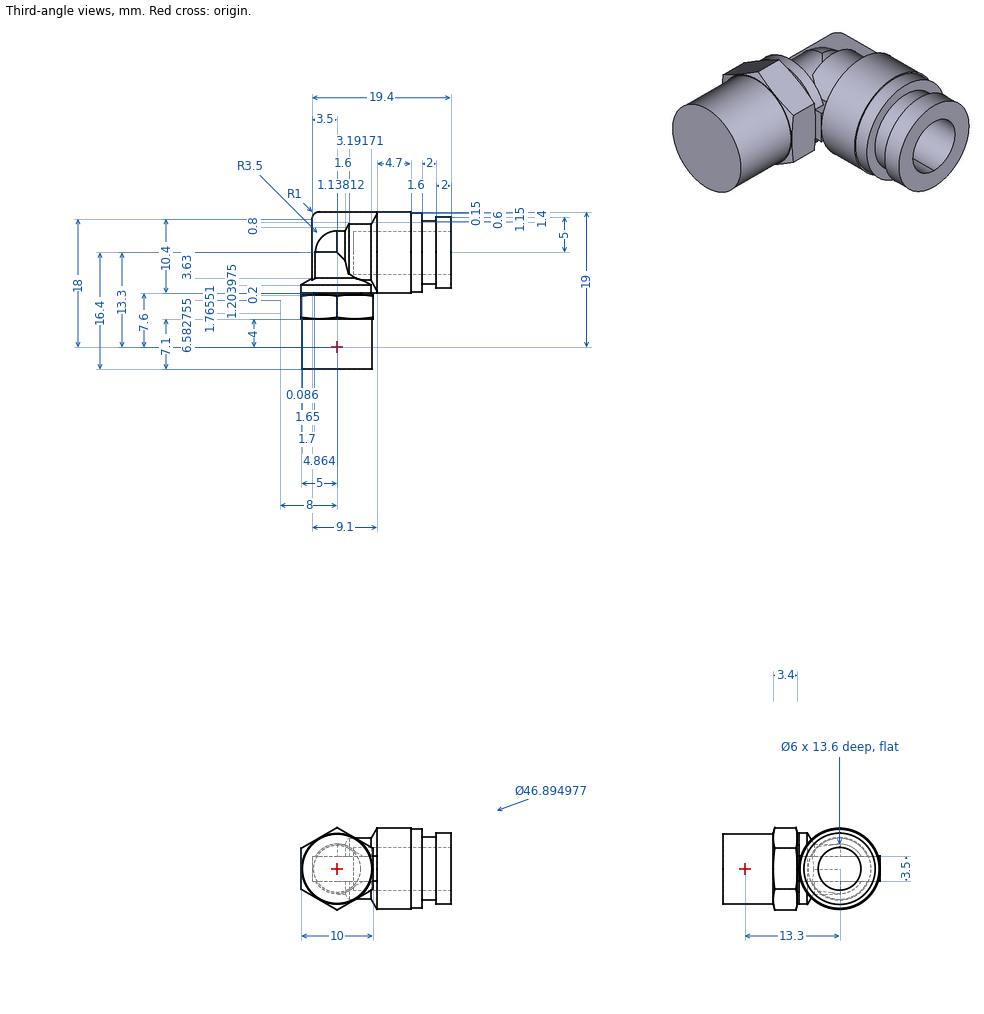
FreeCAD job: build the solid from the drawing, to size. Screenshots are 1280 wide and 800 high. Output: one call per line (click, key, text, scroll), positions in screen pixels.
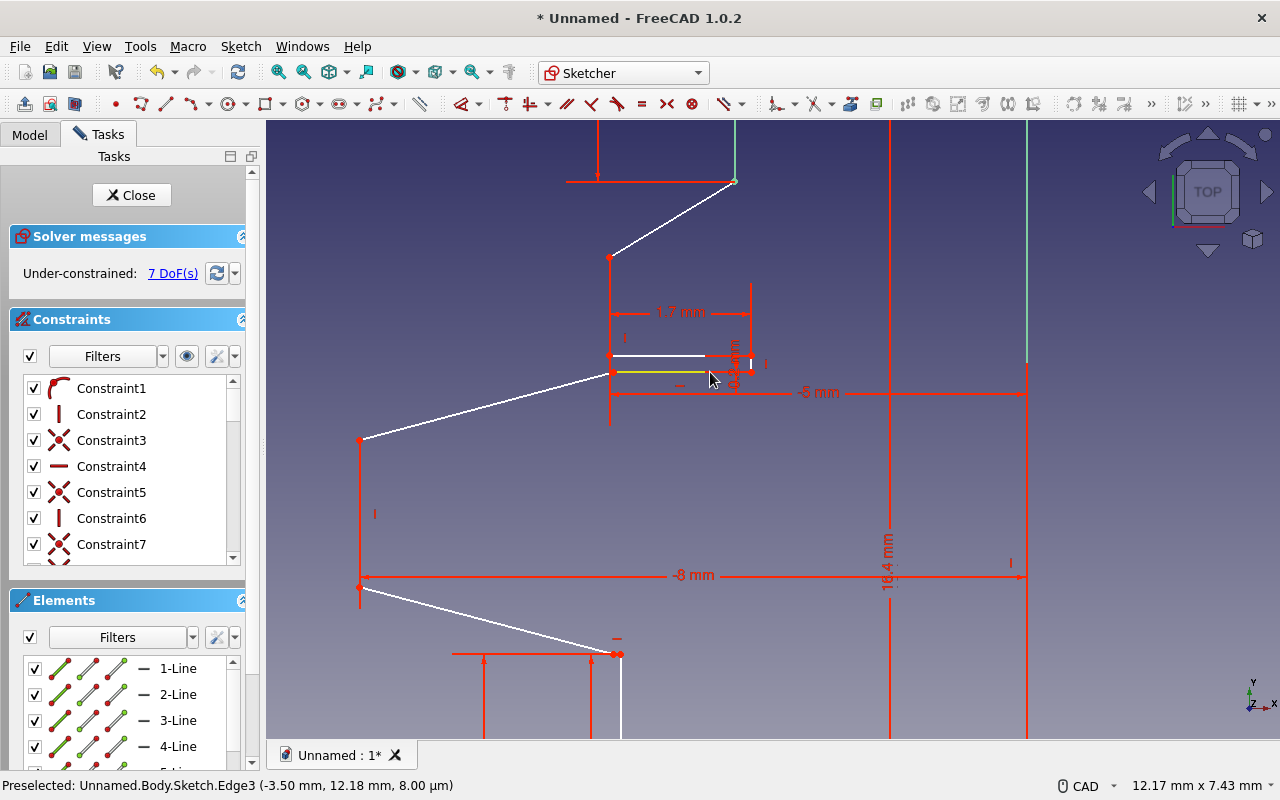
click(710, 372)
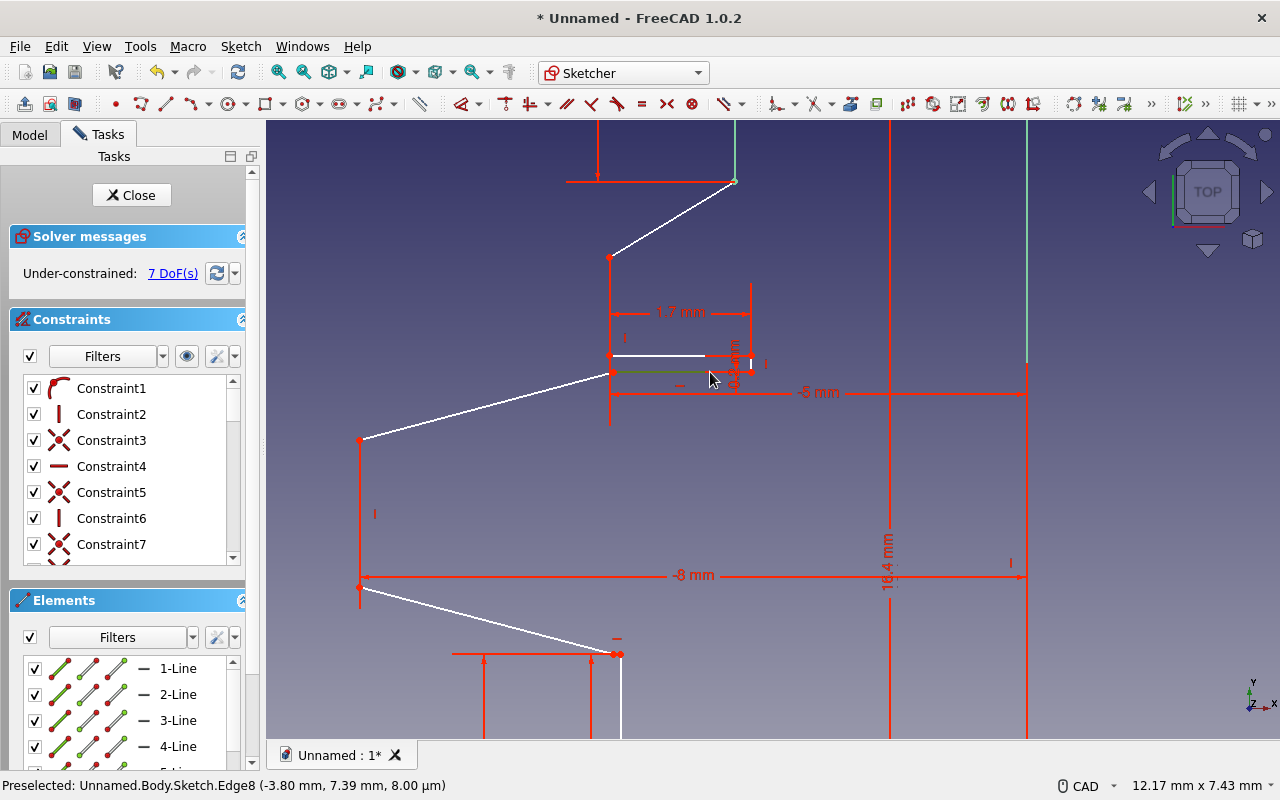
key(l)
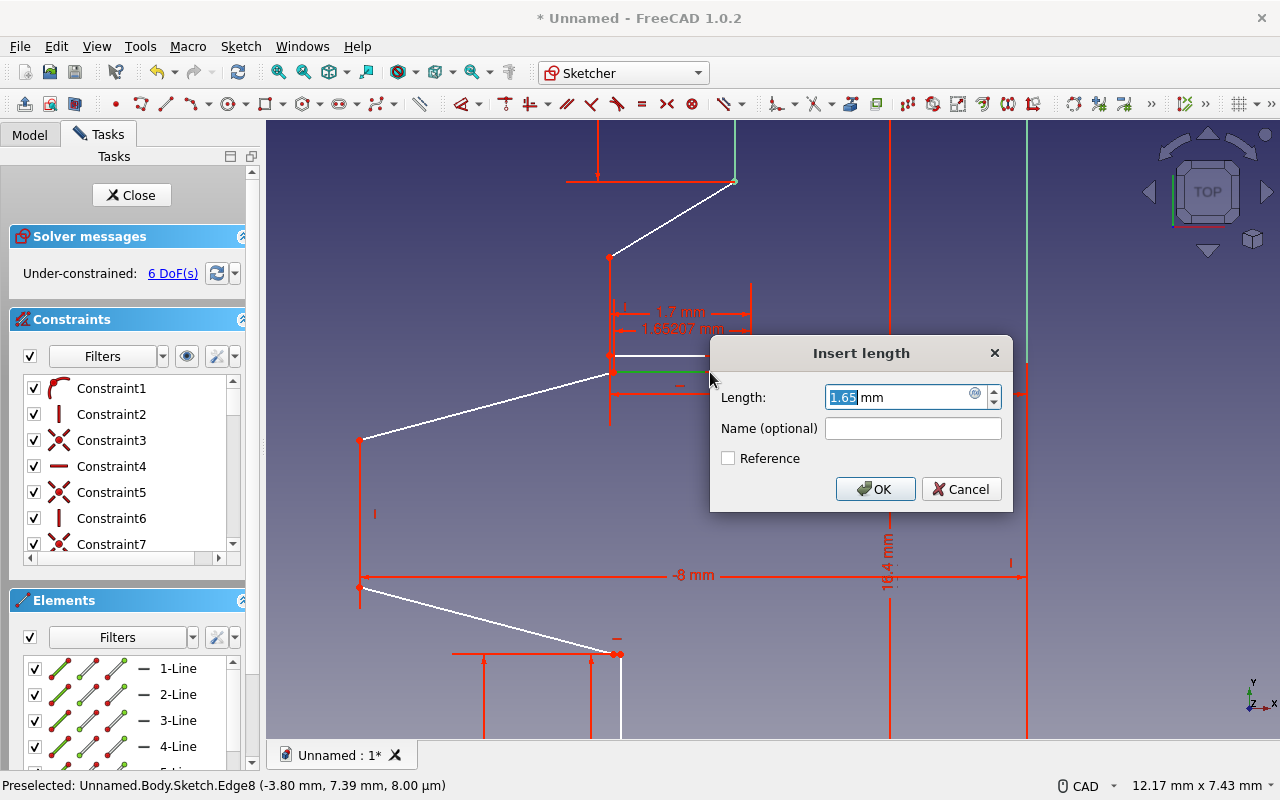
text(1.65)
key(Return)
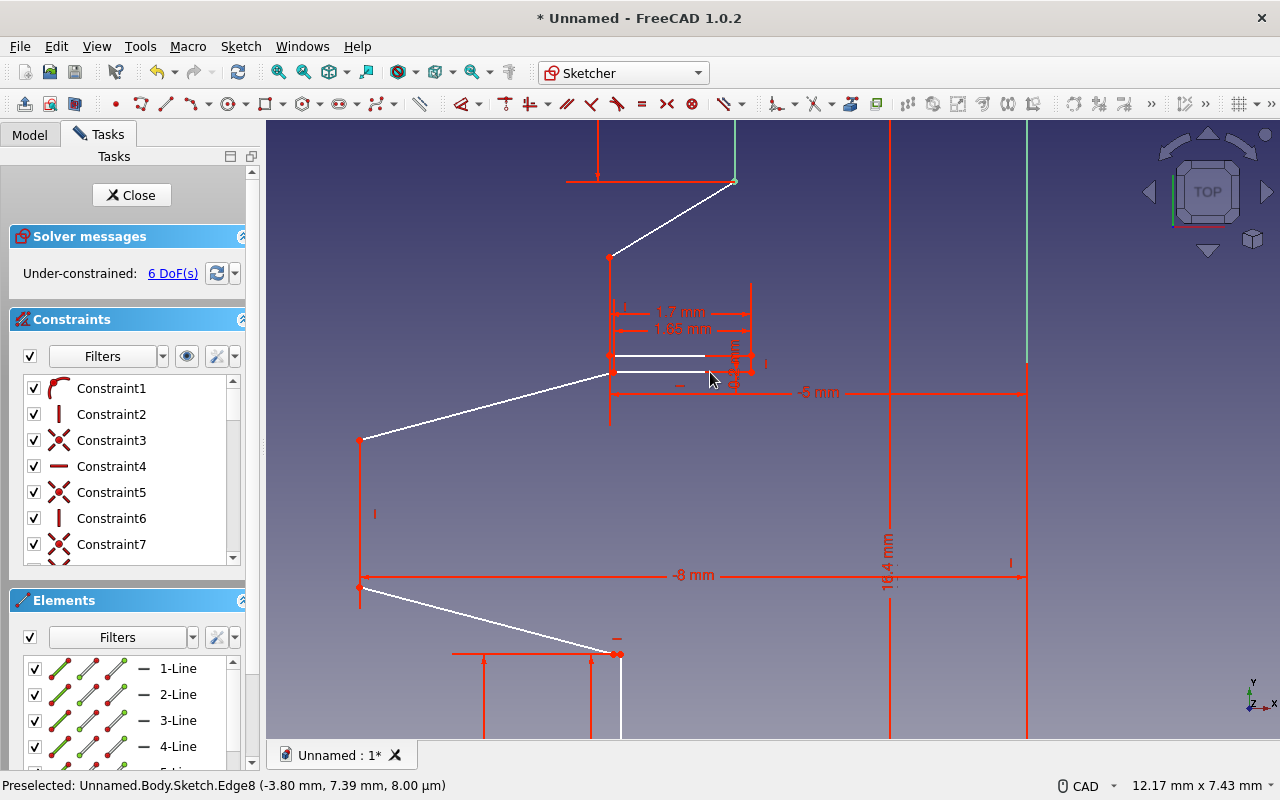
click(610, 356)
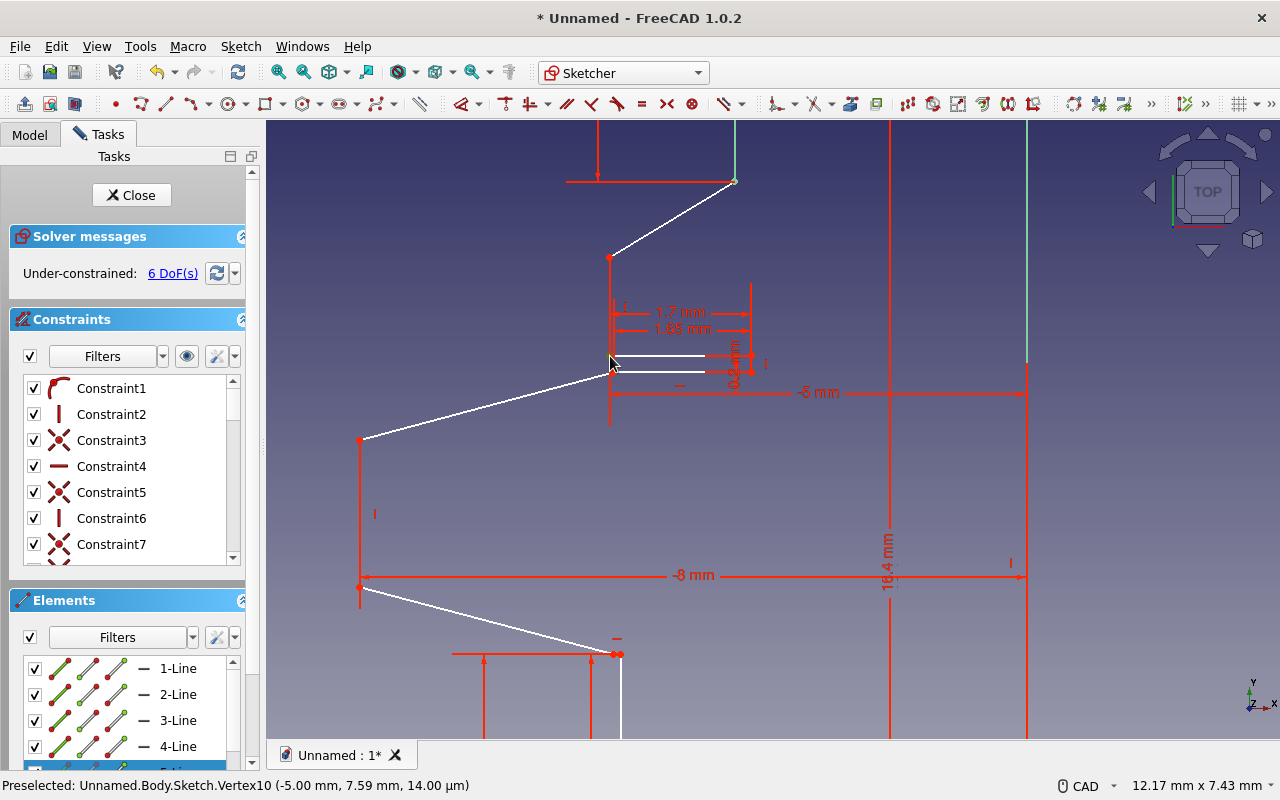
key(i)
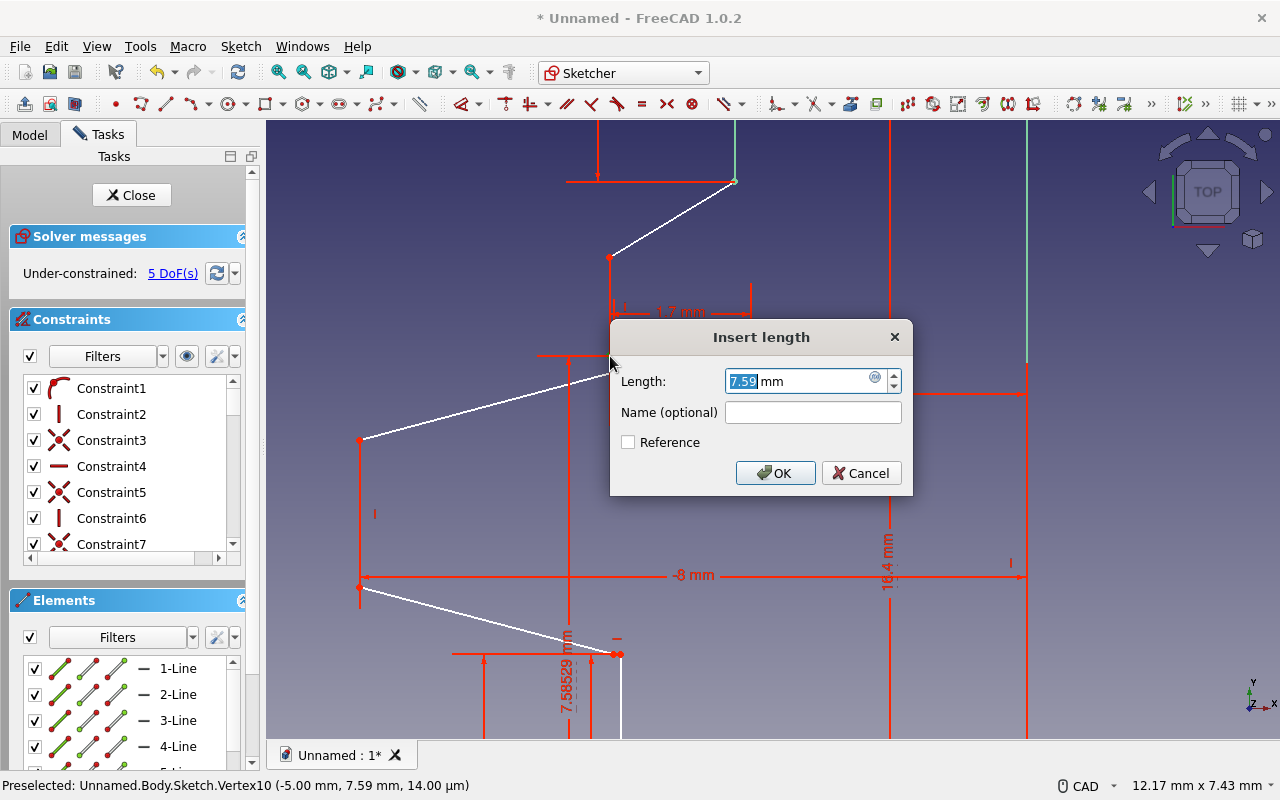
text(7.6)
key(Return)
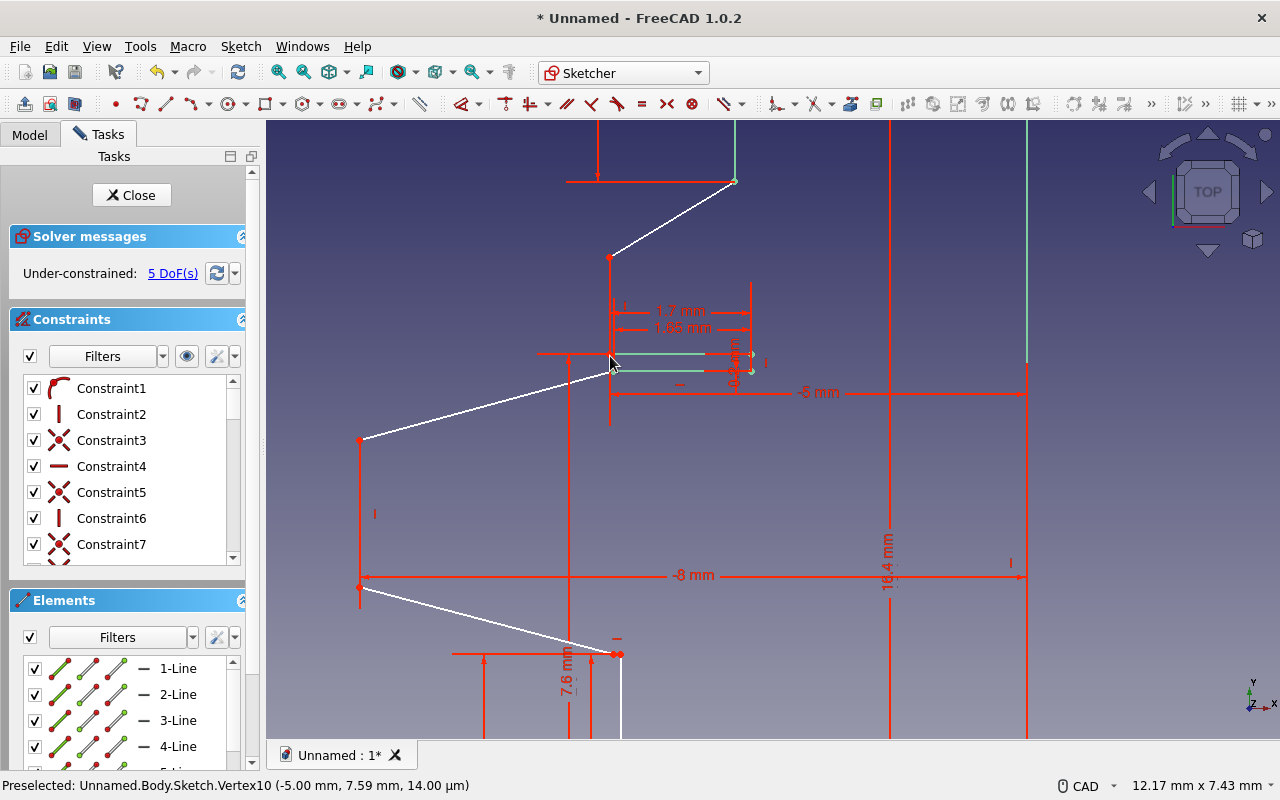
scroll(617, 654, up, 9)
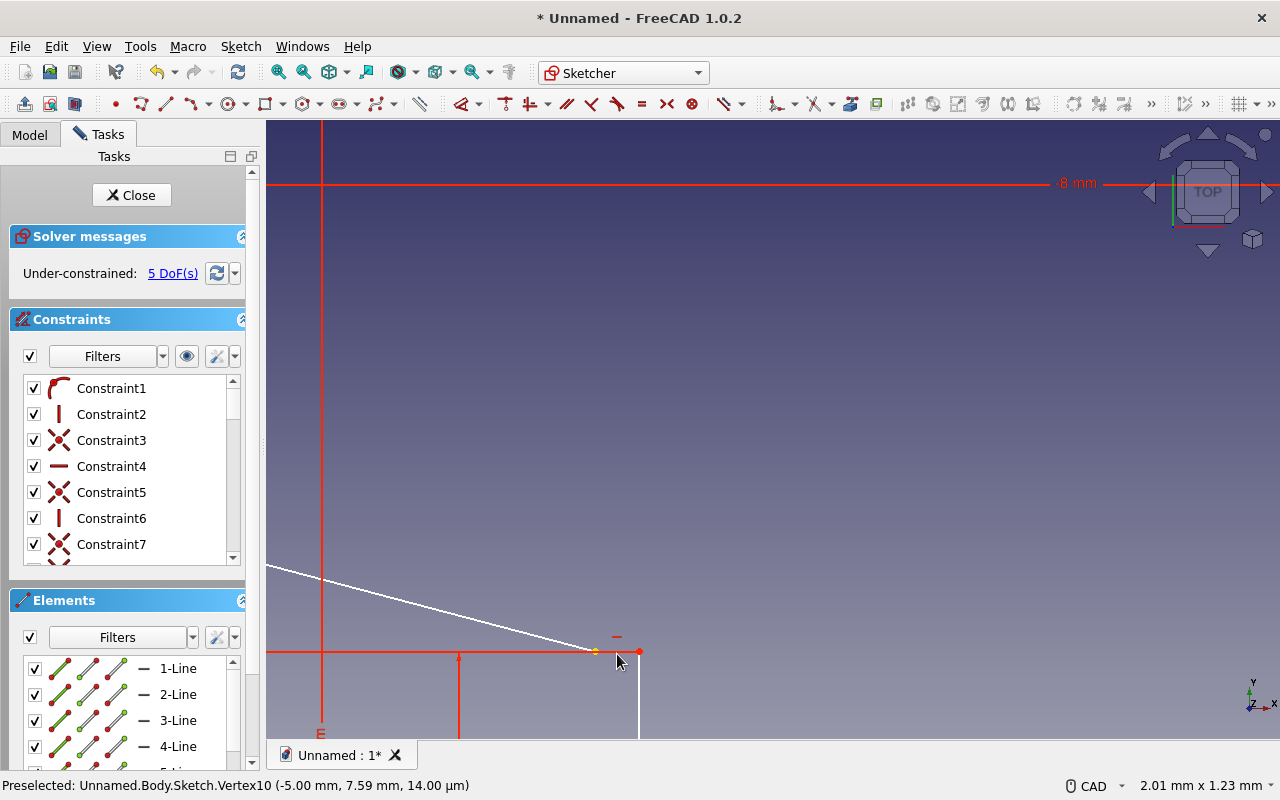
click(618, 652)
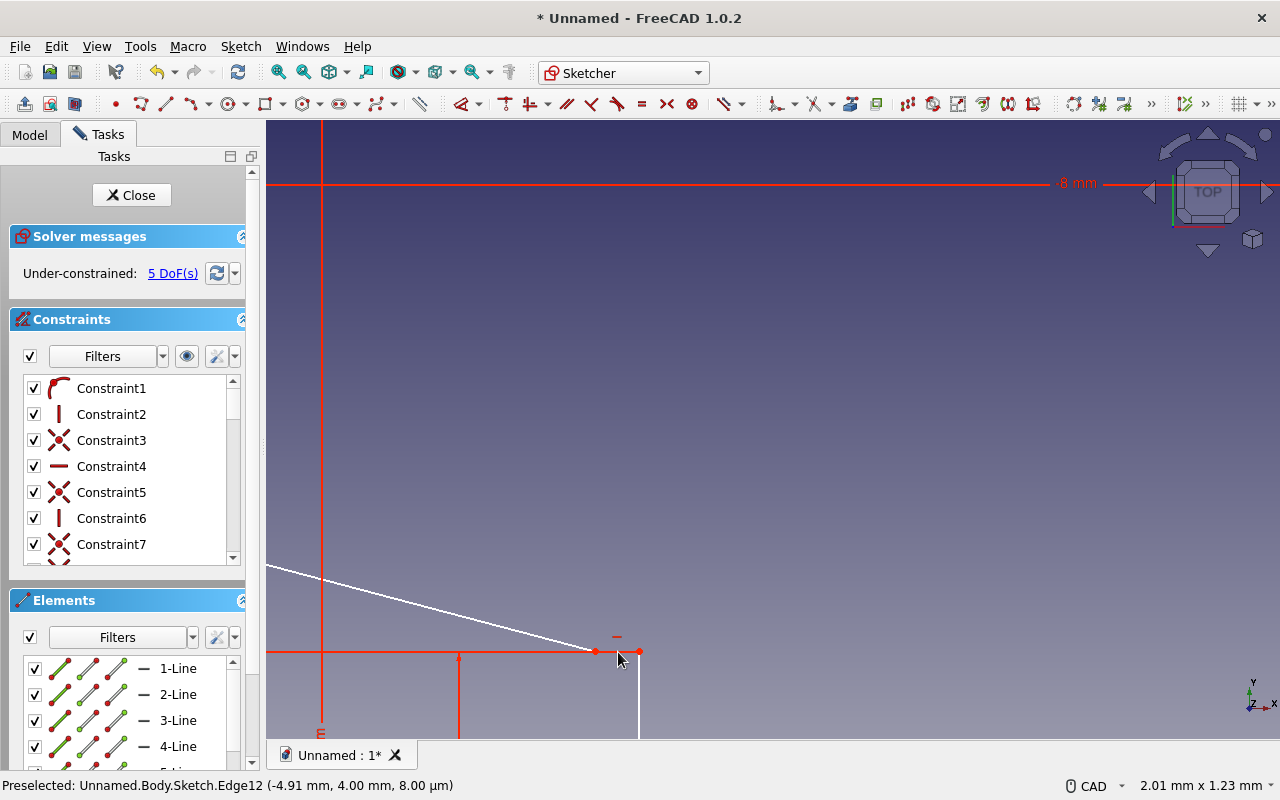
key(l)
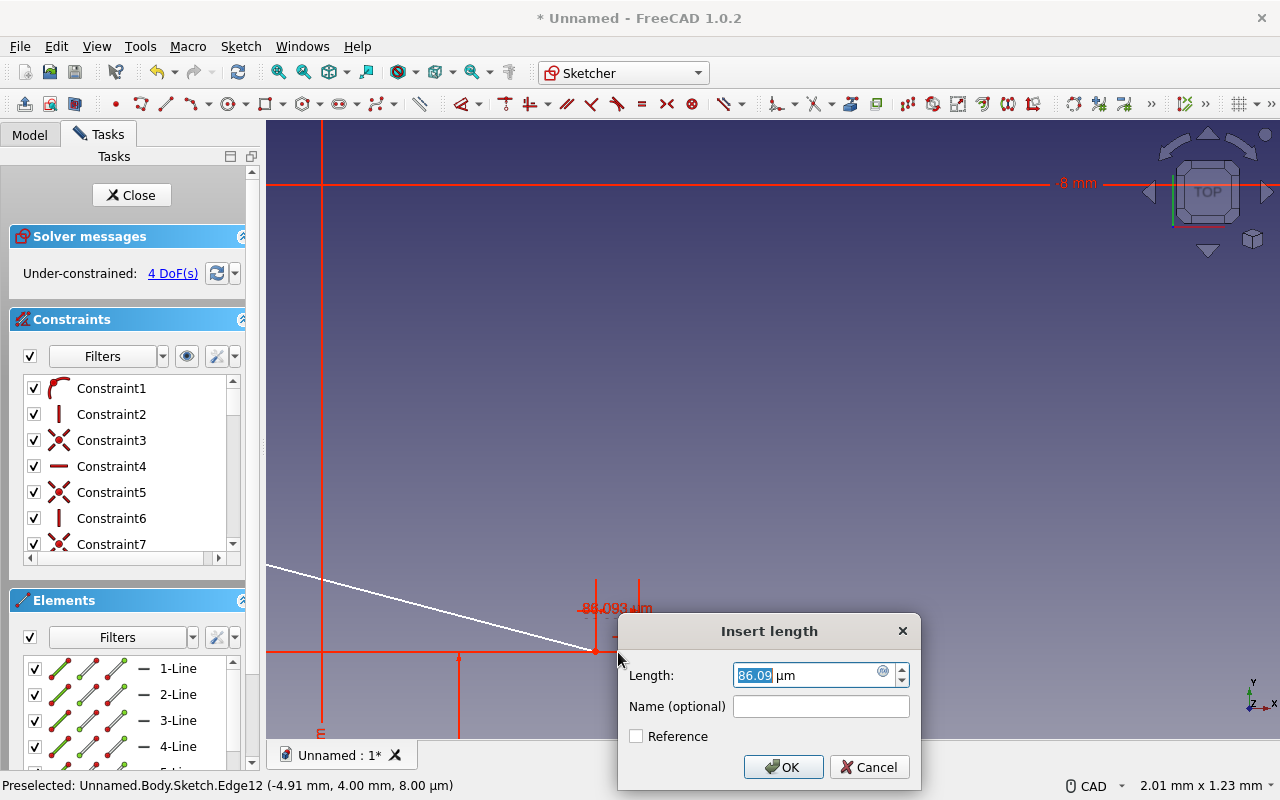
key(ctrl+a)
text(0.086 mm)
key(Return)